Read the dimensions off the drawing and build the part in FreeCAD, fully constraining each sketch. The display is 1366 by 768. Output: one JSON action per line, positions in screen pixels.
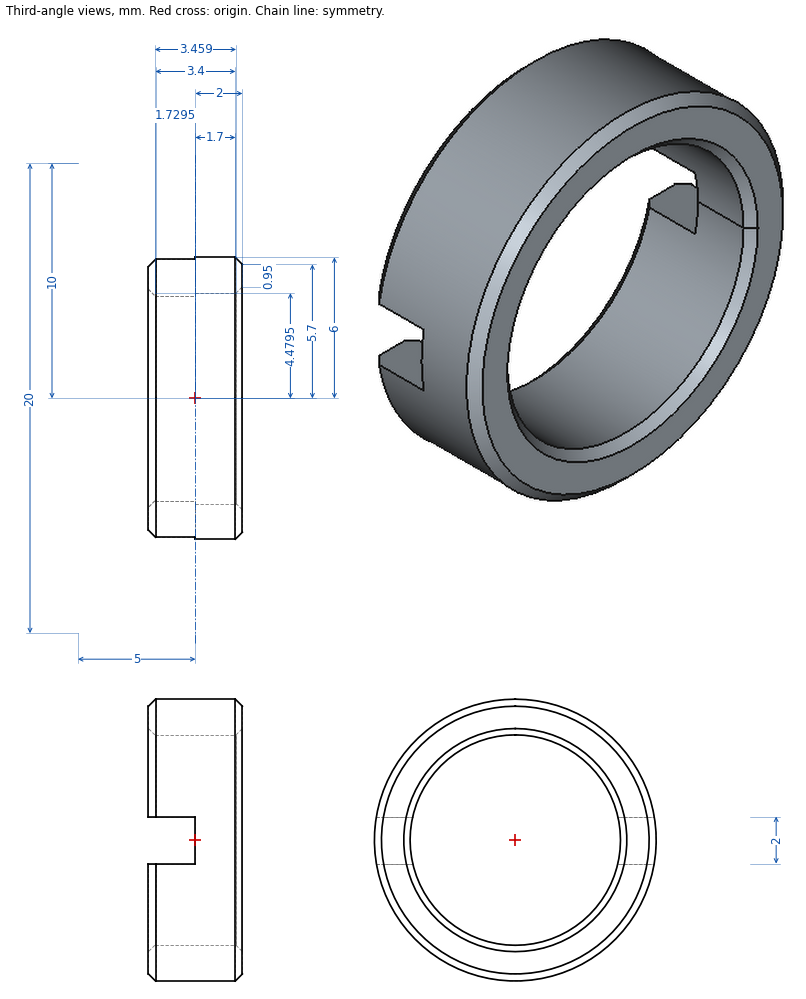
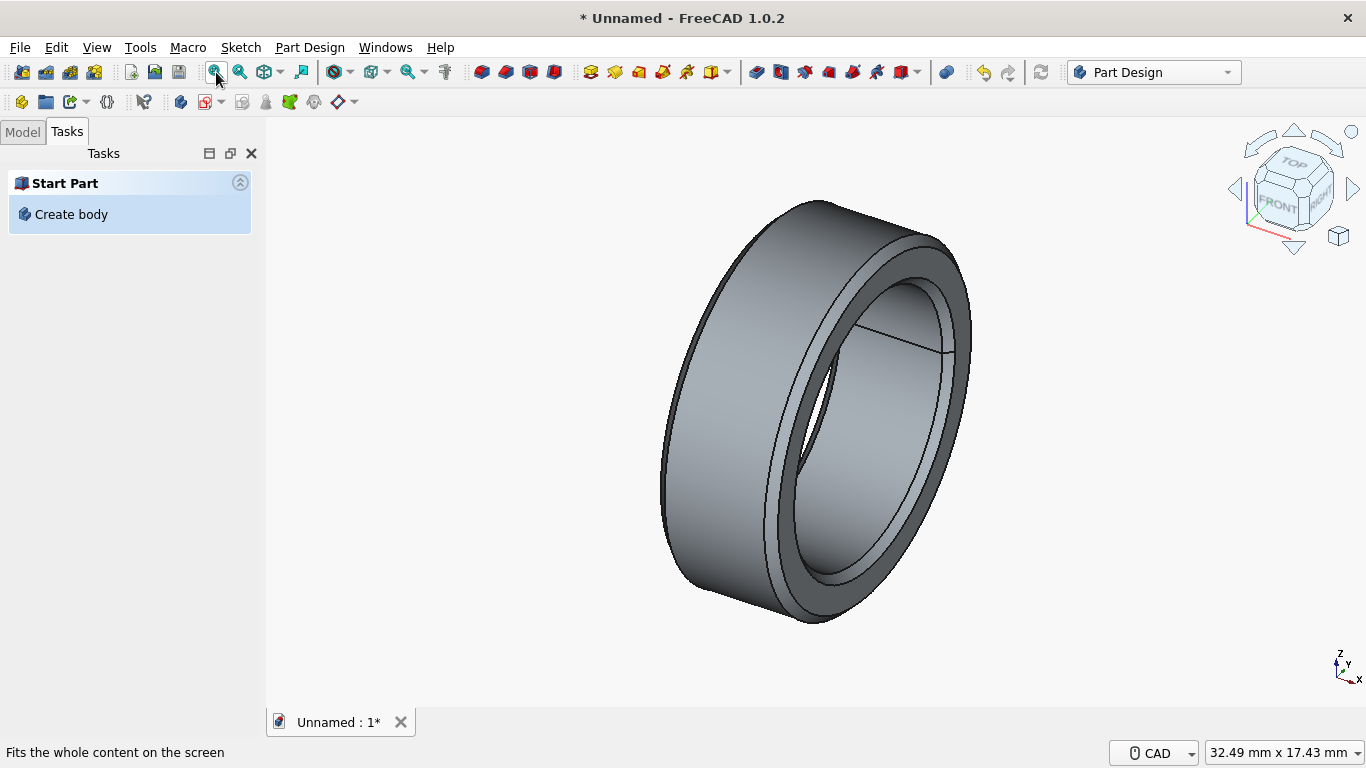
{"action": "left_click", "coordinate": [206, 102]}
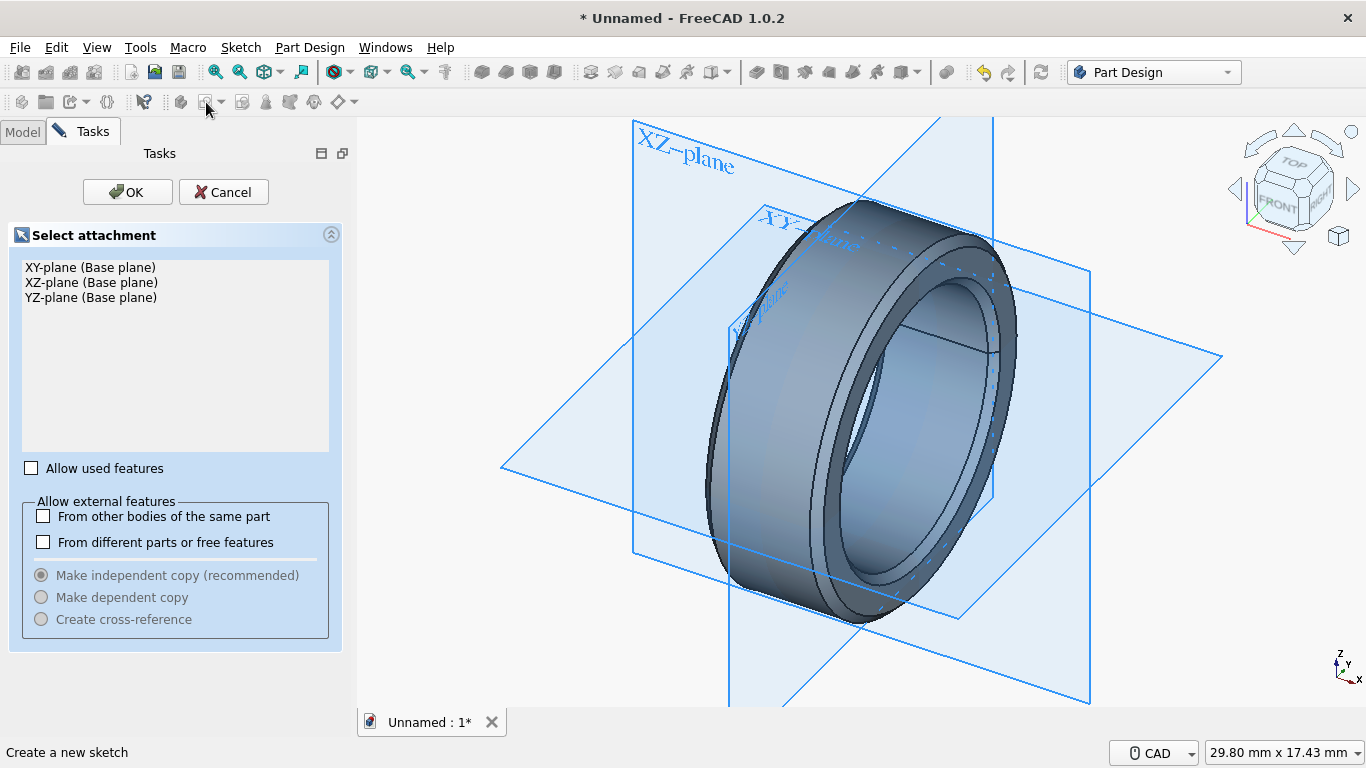
{"action": "left_click", "coordinate": [82, 268]}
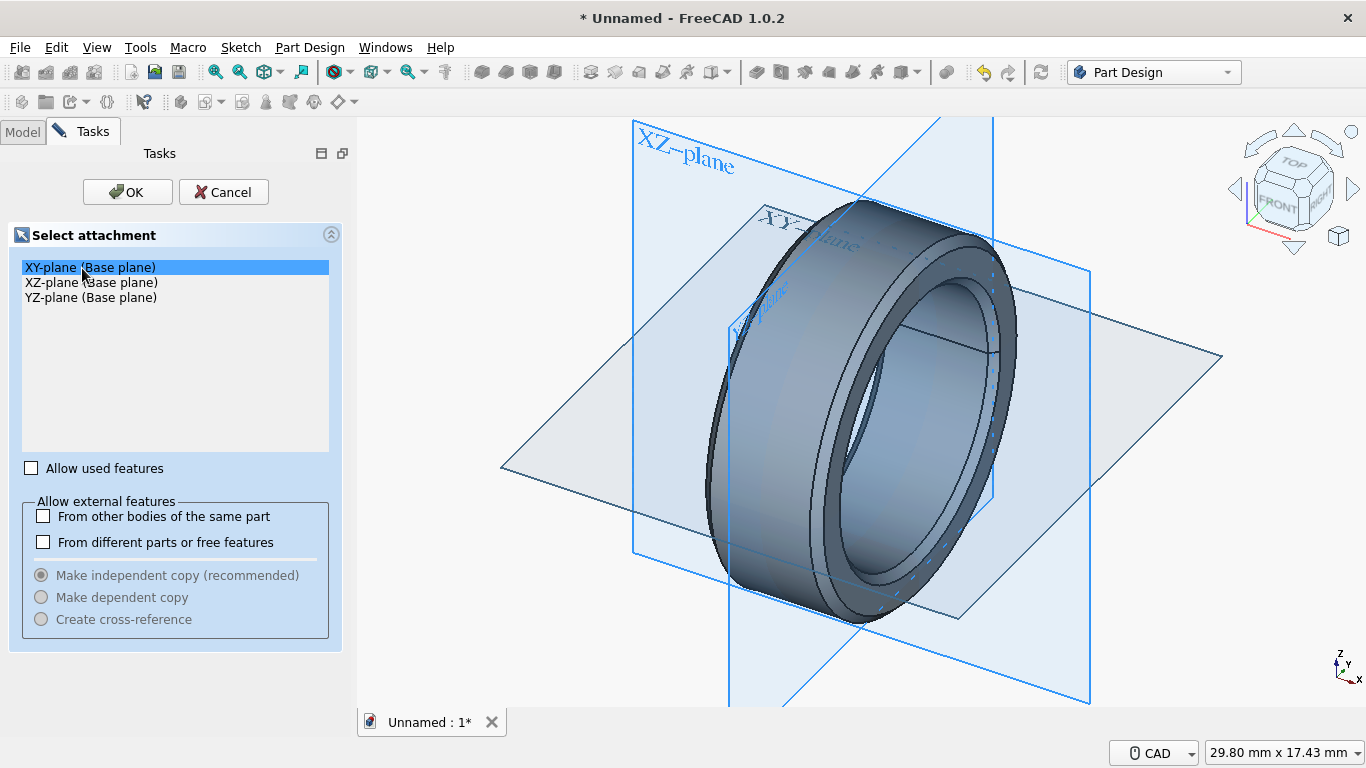
{"action": "left_click", "coordinate": [128, 192]}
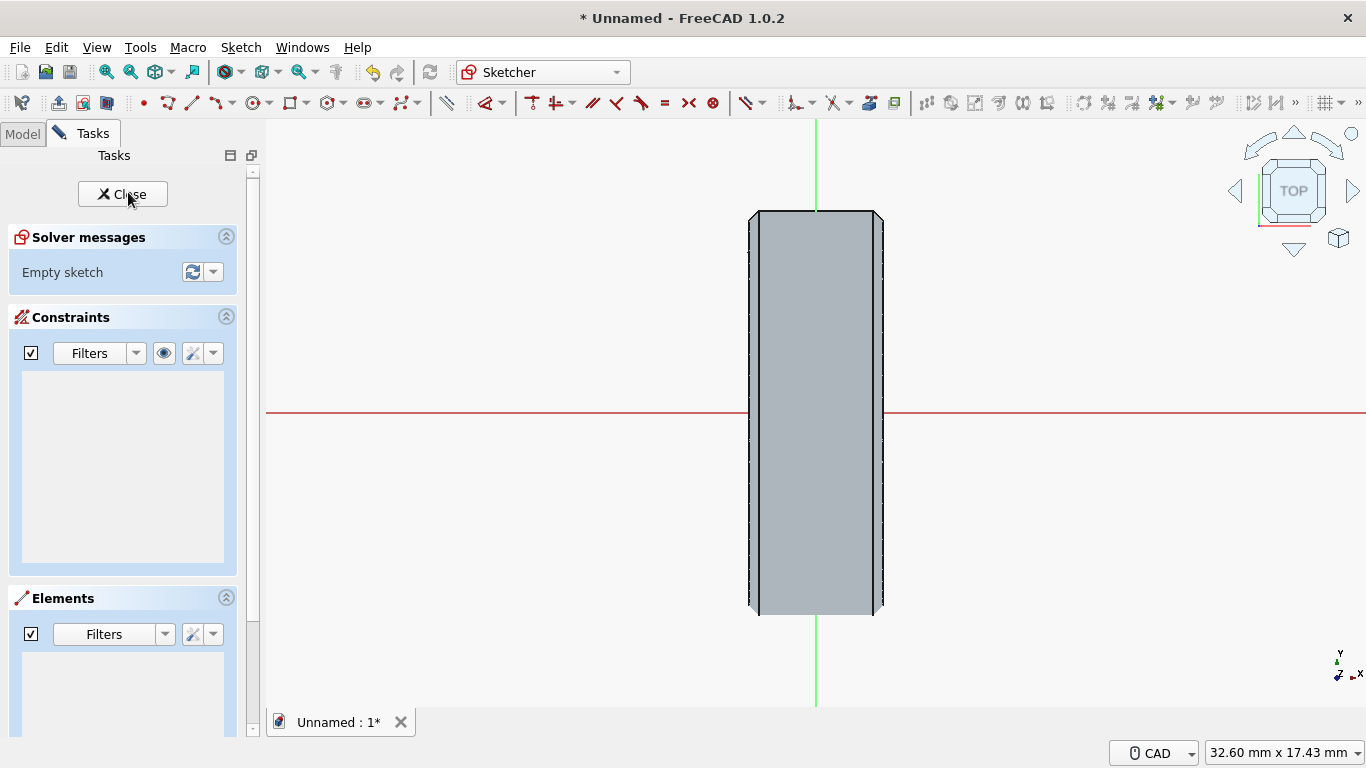
{"action": "left_click", "coordinate": [108, 104]}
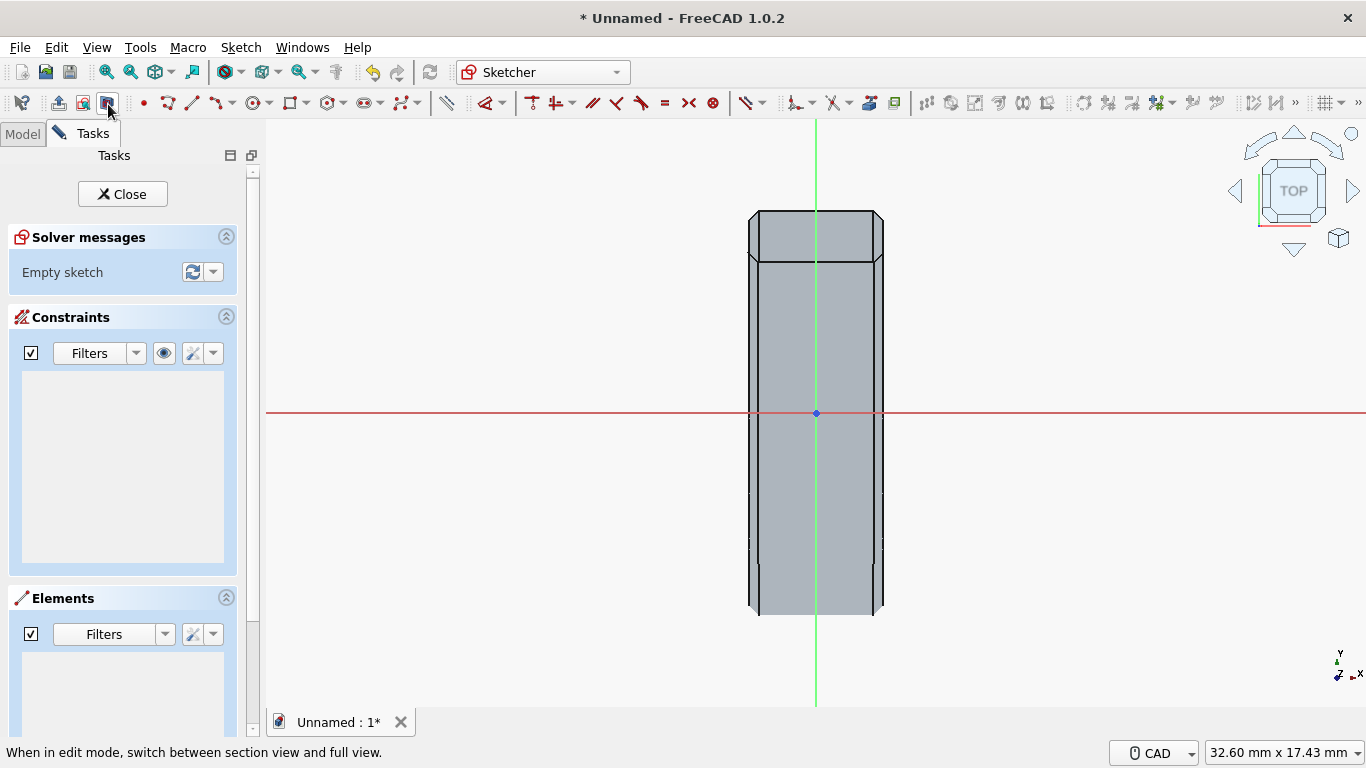
{"action": "scroll", "coordinate": [767, 413], "scroll_direction": "down", "scroll_amount": 3}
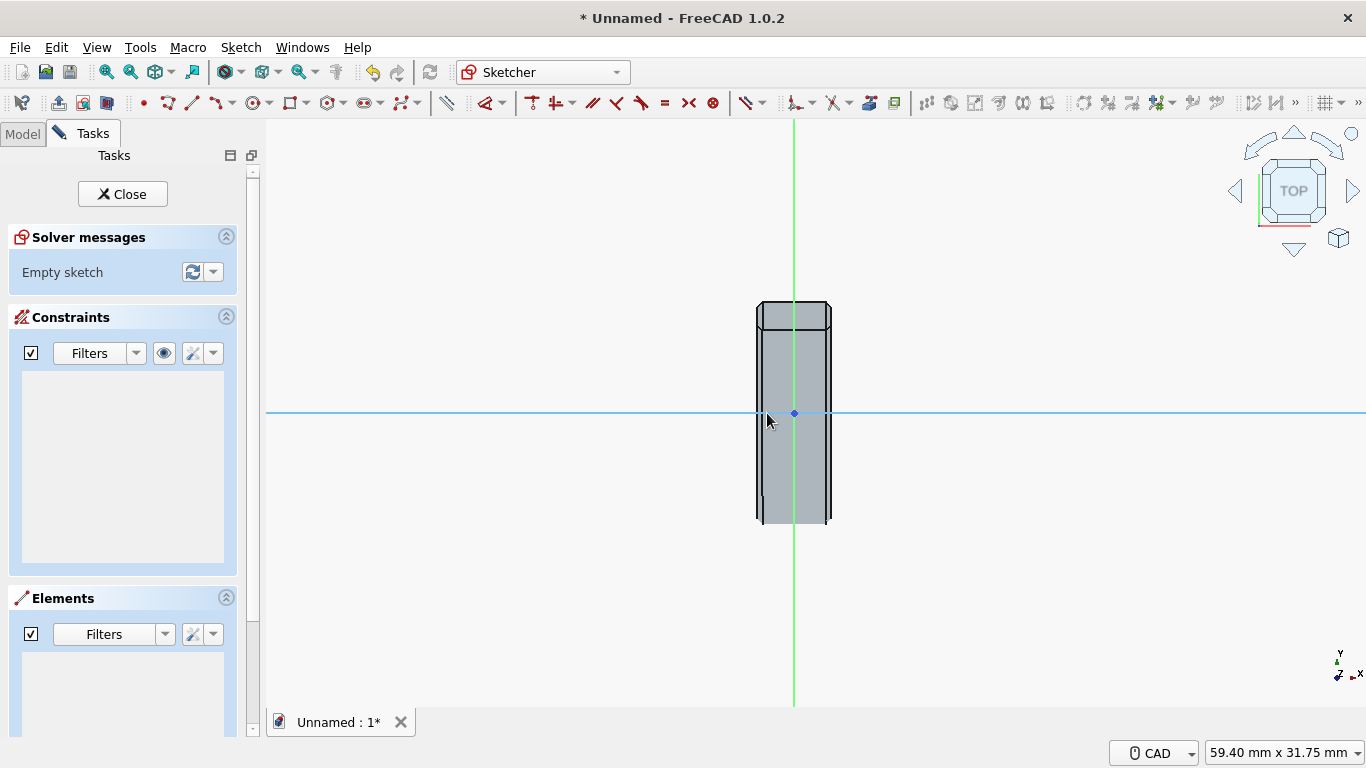
{"action": "left_click", "coordinate": [290, 104]}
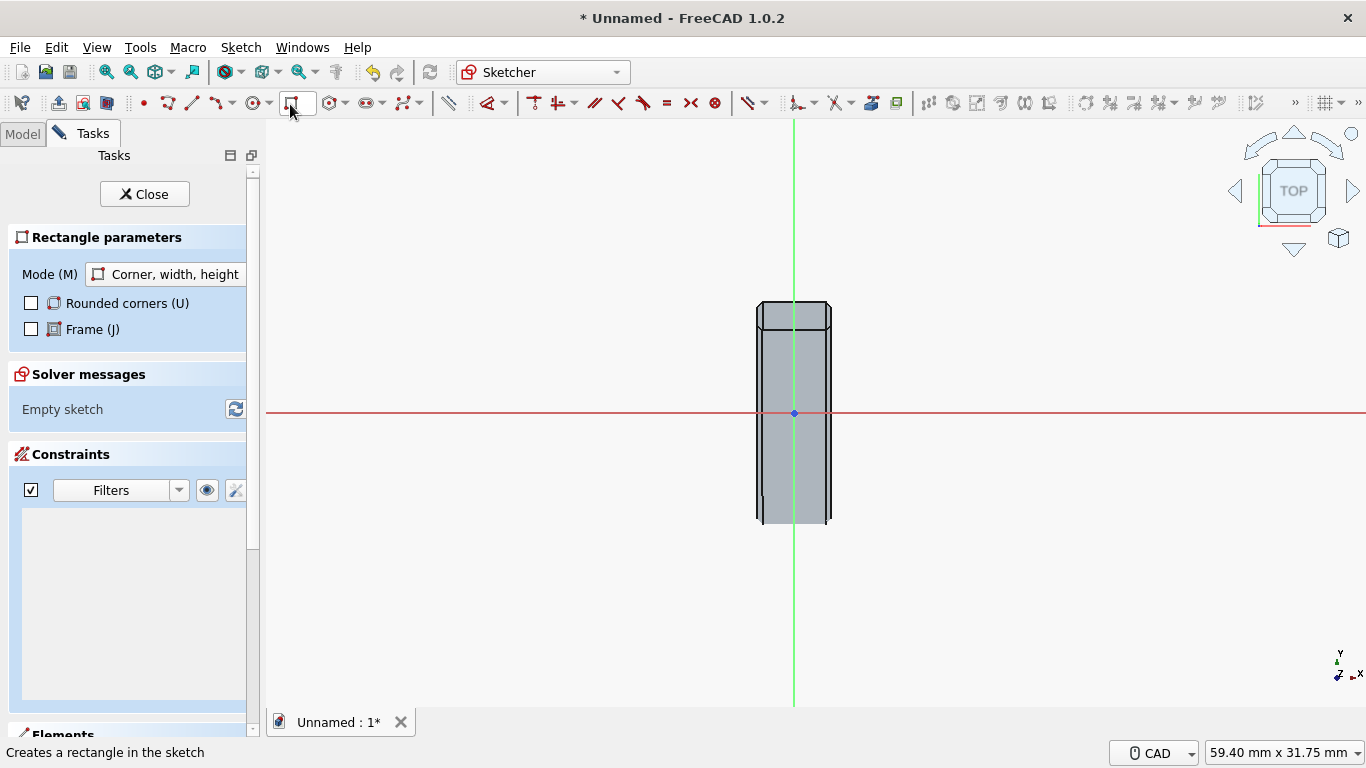
{"action": "left_click", "coordinate": [702, 228]}
{"action": "left_click", "coordinate": [794, 598]}
{"action": "key", "text": "Escape"}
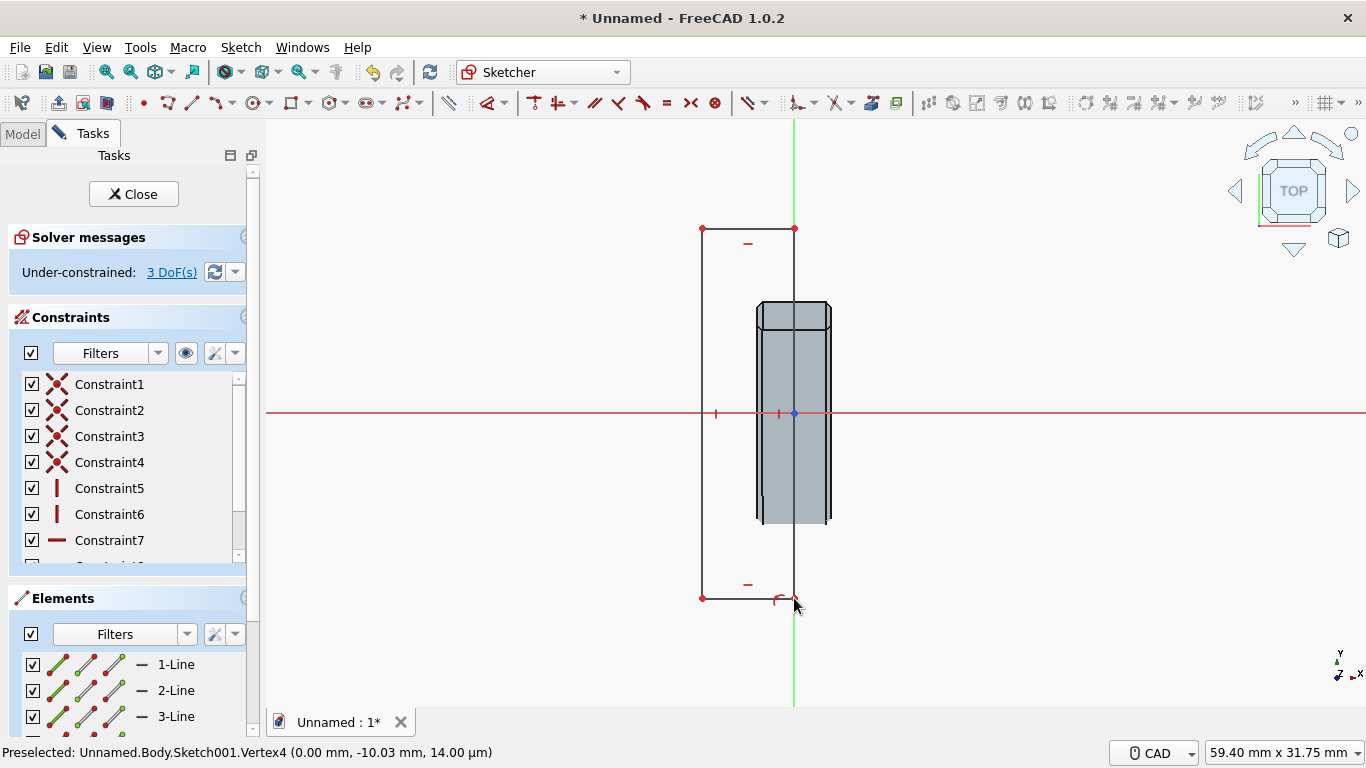
{"action": "left_click", "coordinate": [488, 104]}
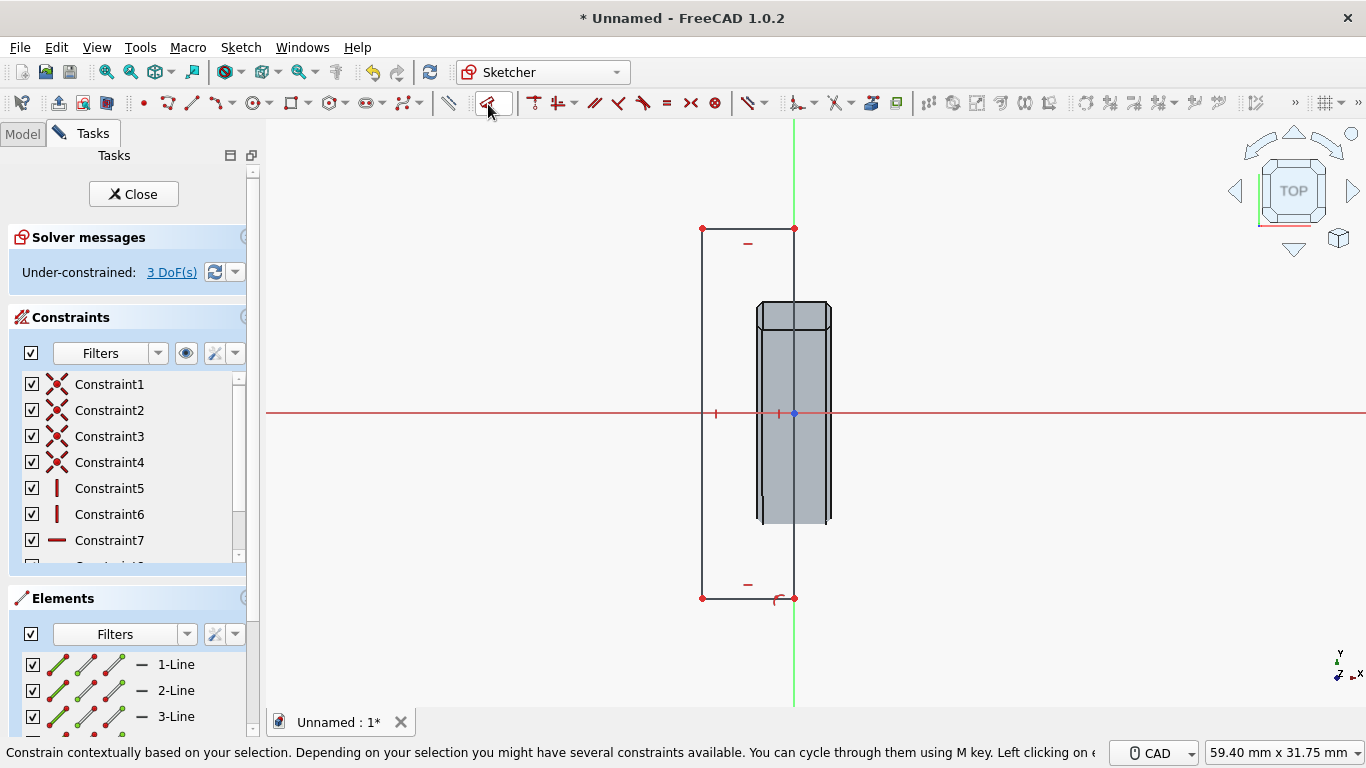
{"action": "left_click", "coordinate": [730, 599]}
{"action": "left_click", "coordinate": [748, 633]}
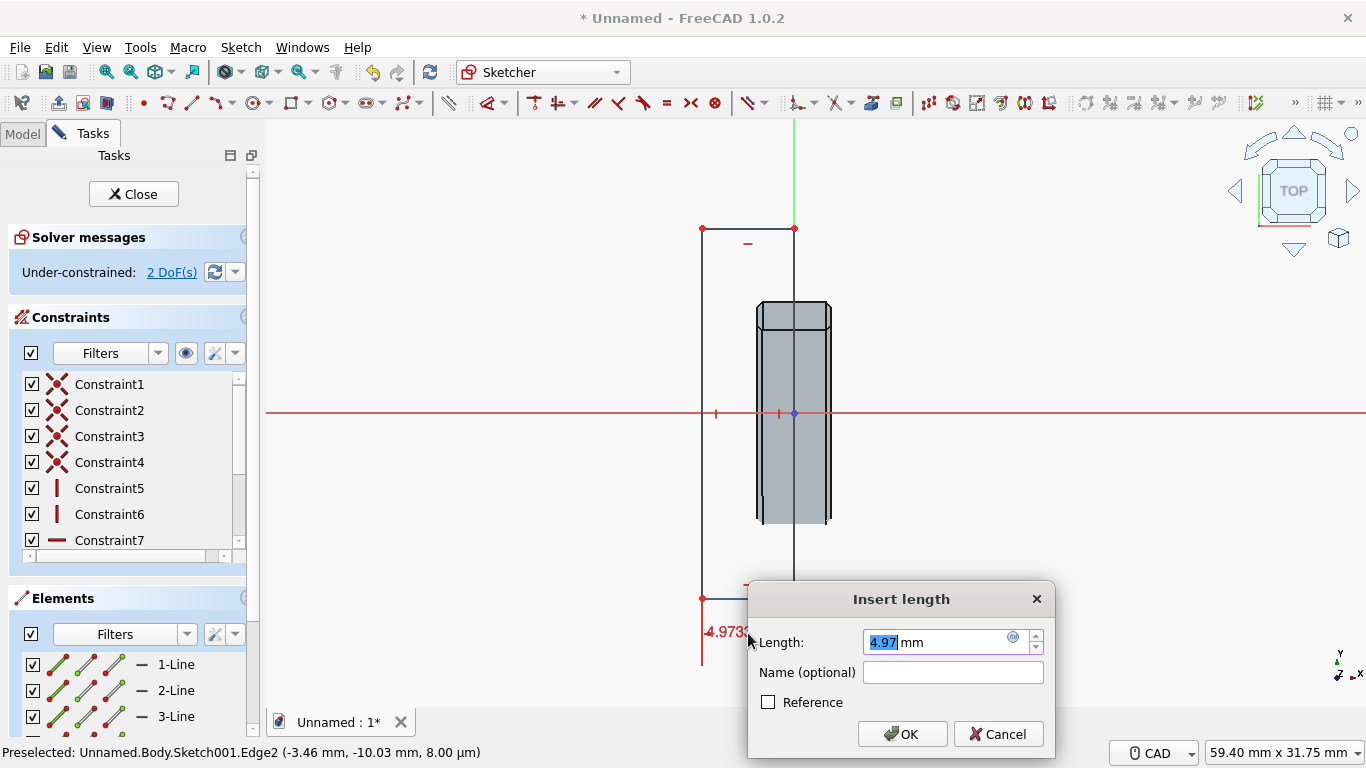
{"action": "type", "text": "5"}
{"action": "key", "text": "Return"}